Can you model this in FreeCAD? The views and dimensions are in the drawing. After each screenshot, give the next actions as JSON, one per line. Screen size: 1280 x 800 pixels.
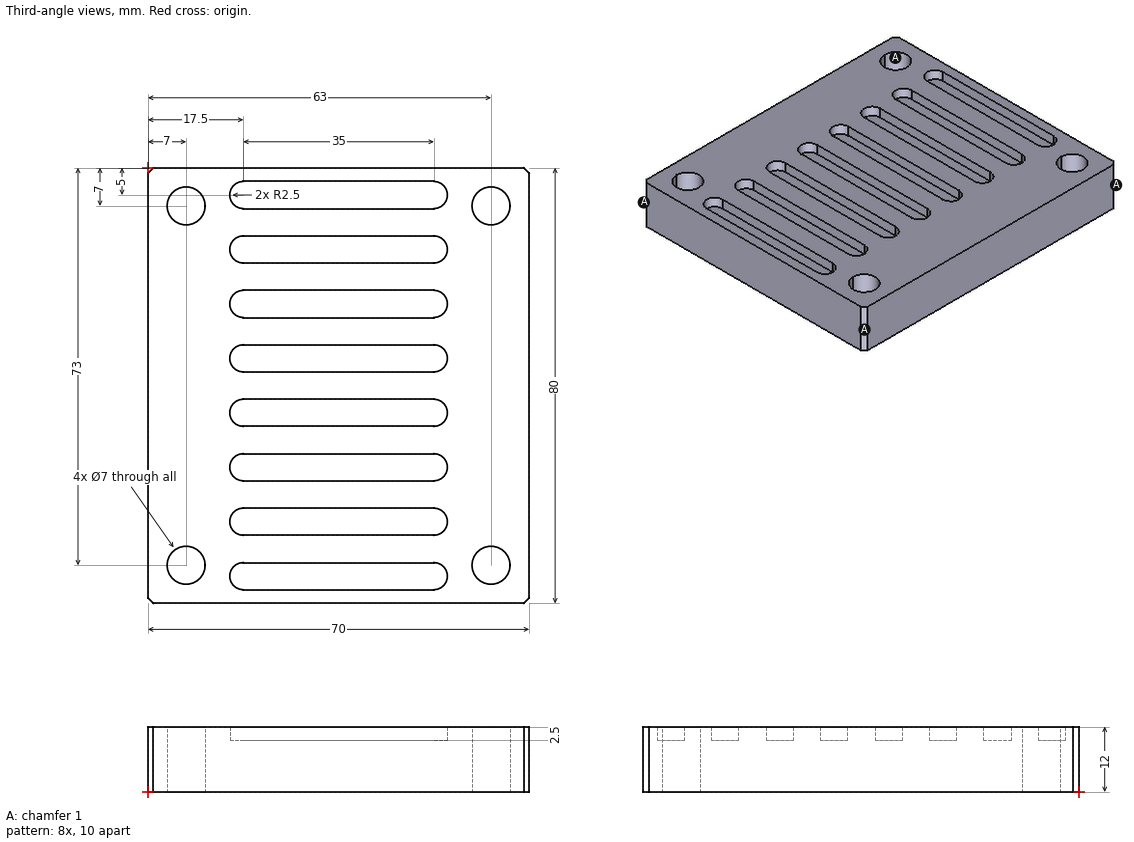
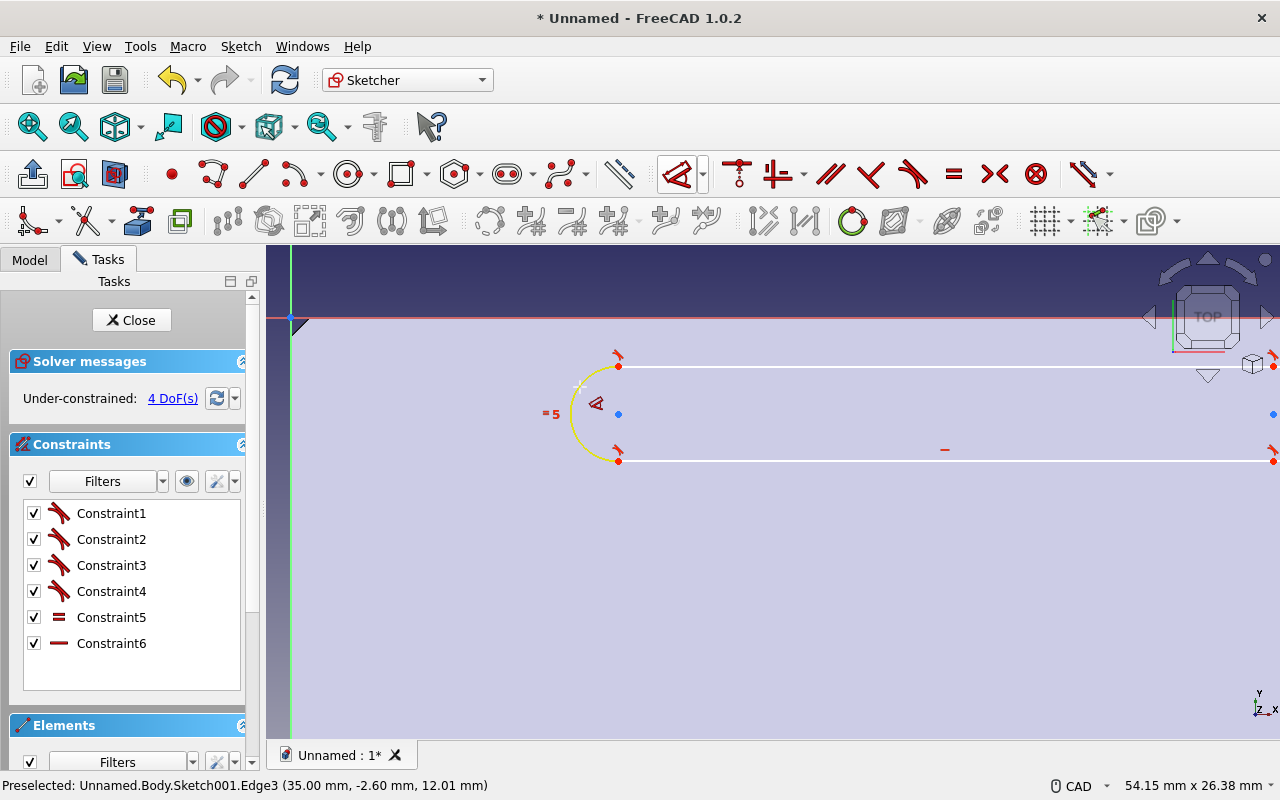
{"action": "left_click", "coordinate": [580, 386]}
{"action": "left_click", "coordinate": [554, 367]}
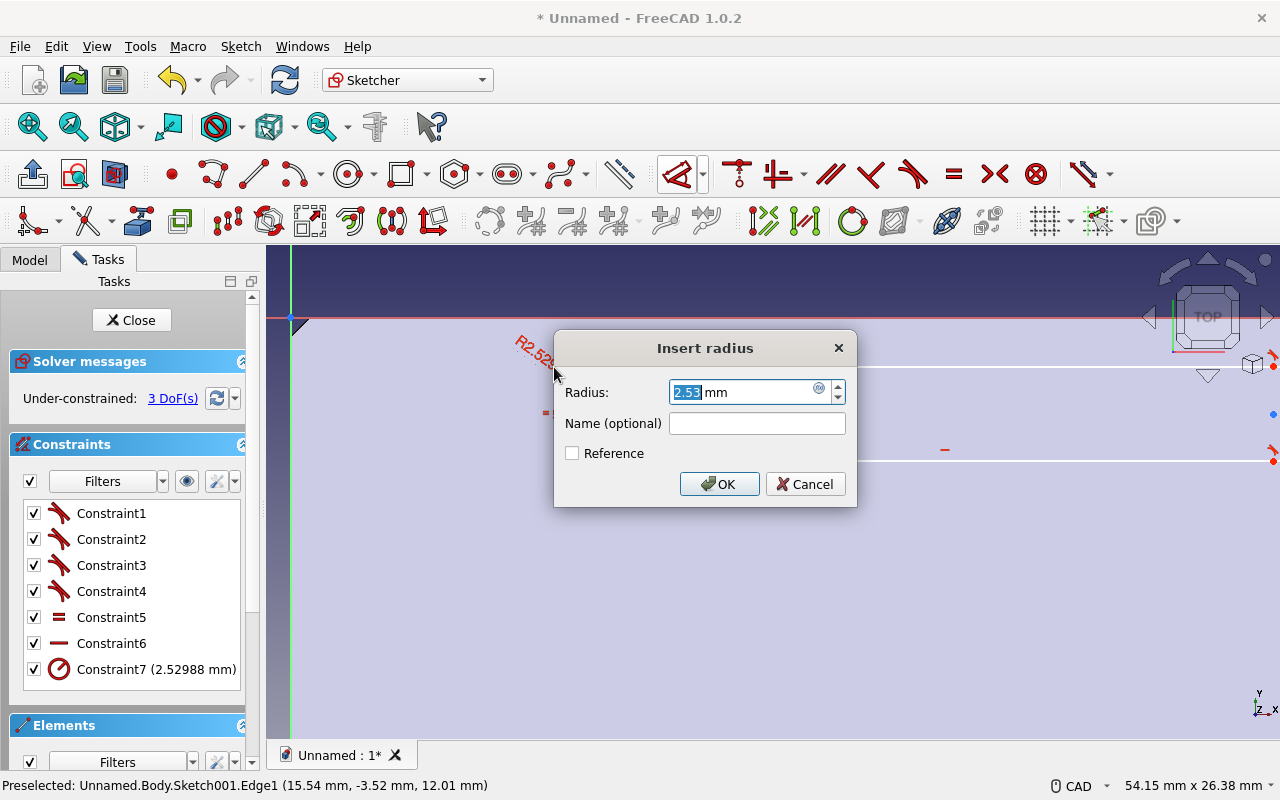
{"action": "type", "text": "2.5"}
{"action": "key", "text": "Return"}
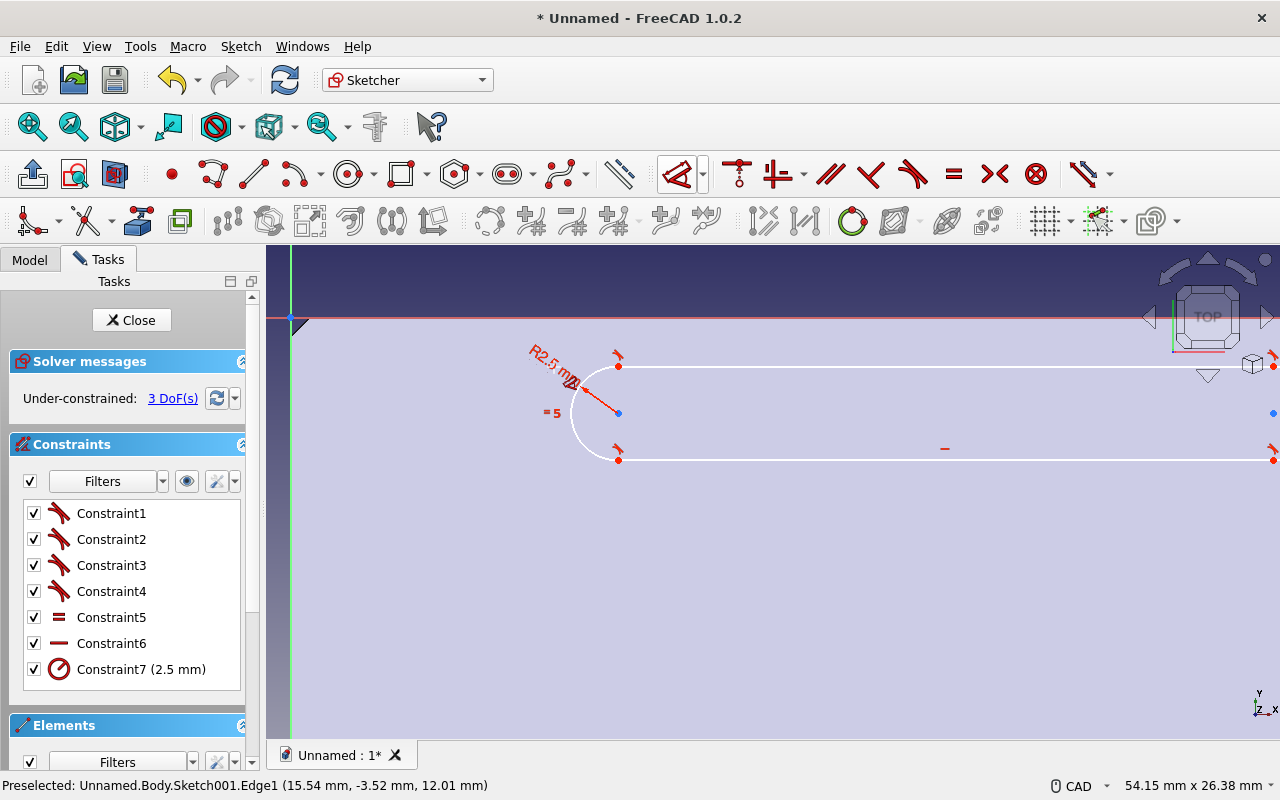
{"action": "left_click", "coordinate": [815, 367]}
{"action": "left_click", "coordinate": [867, 333]}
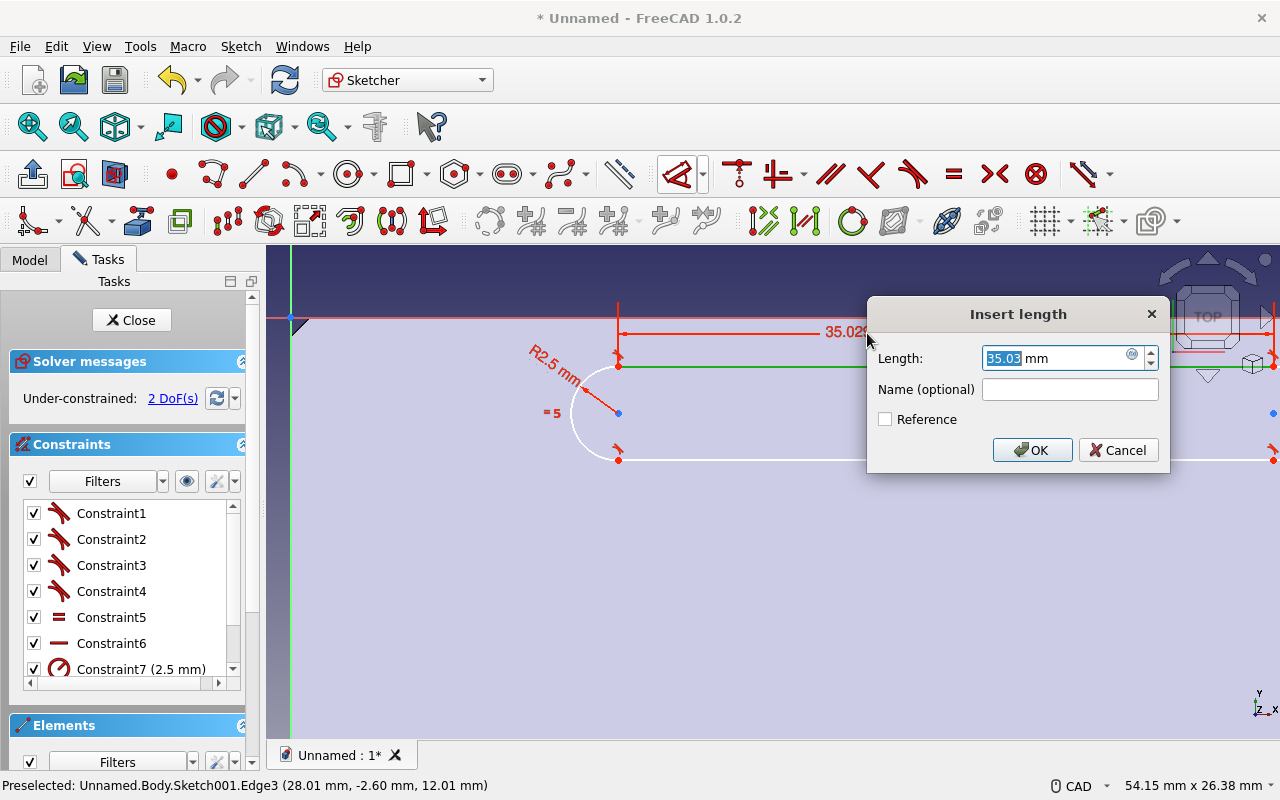
{"action": "type", "text": "35"}
{"action": "key", "text": "Return"}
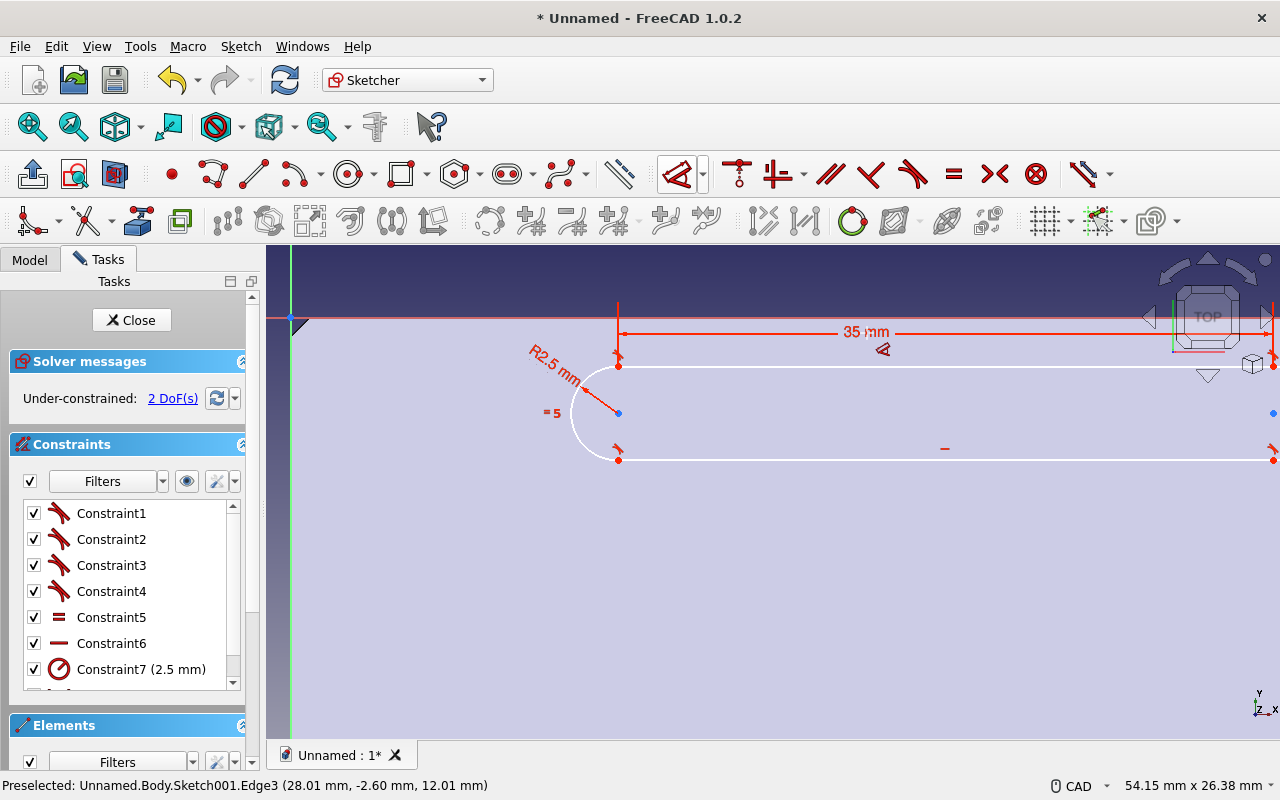
{"action": "left_click", "coordinate": [618, 414]}
{"action": "left_click", "coordinate": [652, 344]}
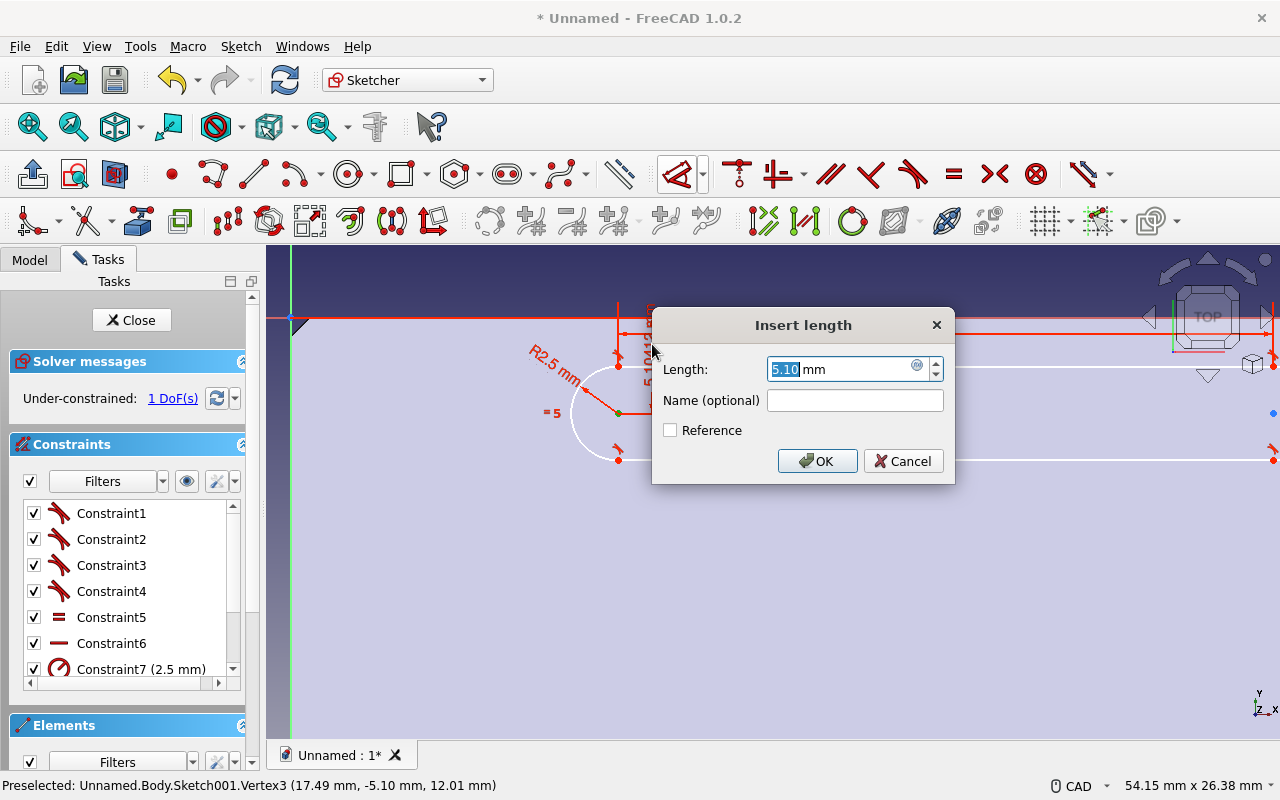
{"action": "type", "text": "5"}
{"action": "key", "text": "Return"}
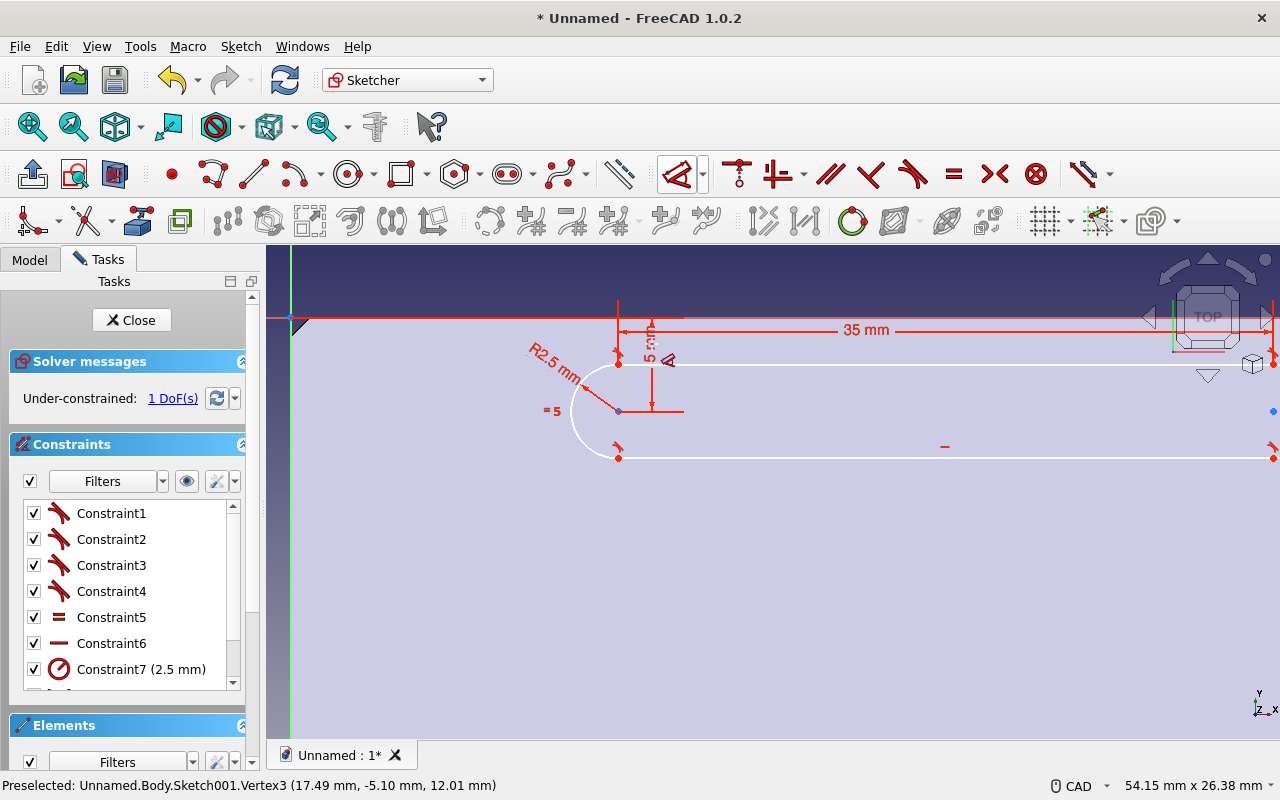
{"action": "left_click", "coordinate": [618, 365]}
{"action": "left_click", "coordinate": [456, 284]}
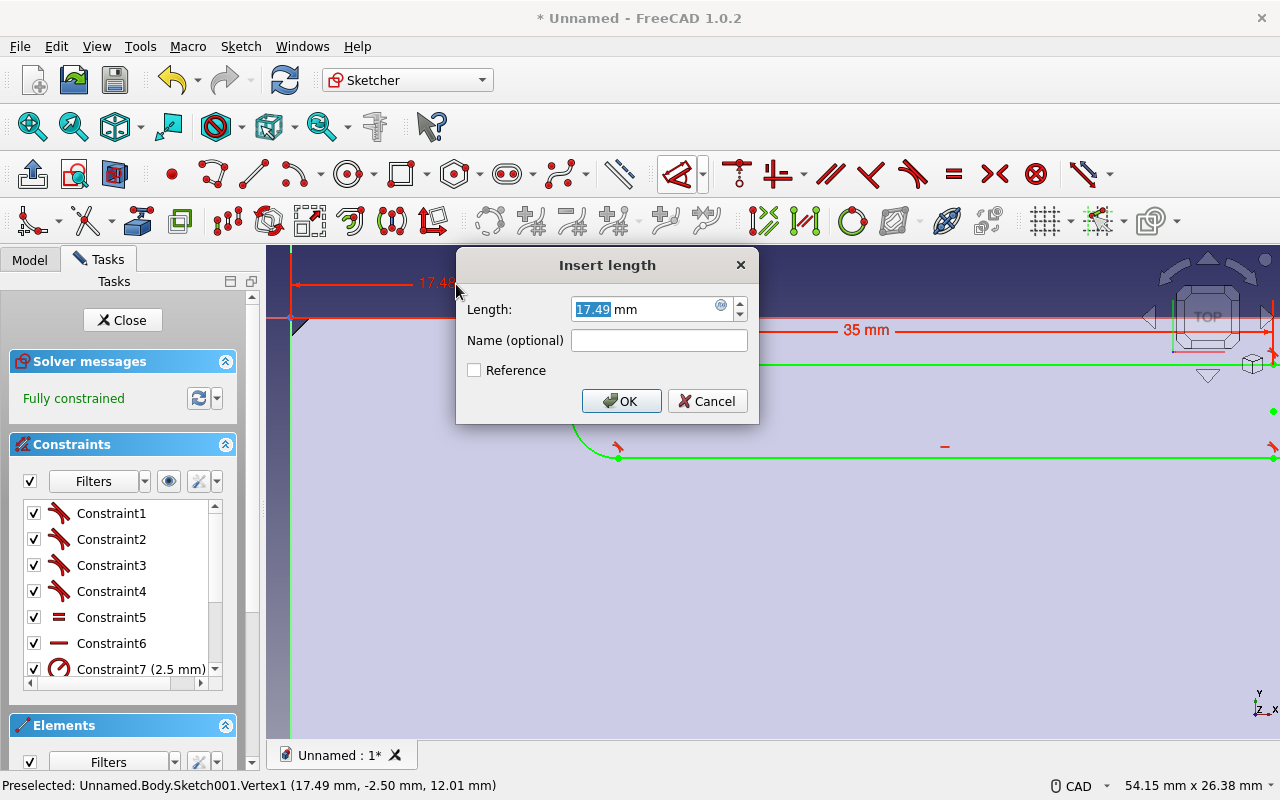
{"action": "type", "text": "17.5"}
{"action": "key", "text": "Return"}
{"action": "key", "text": "Escape"}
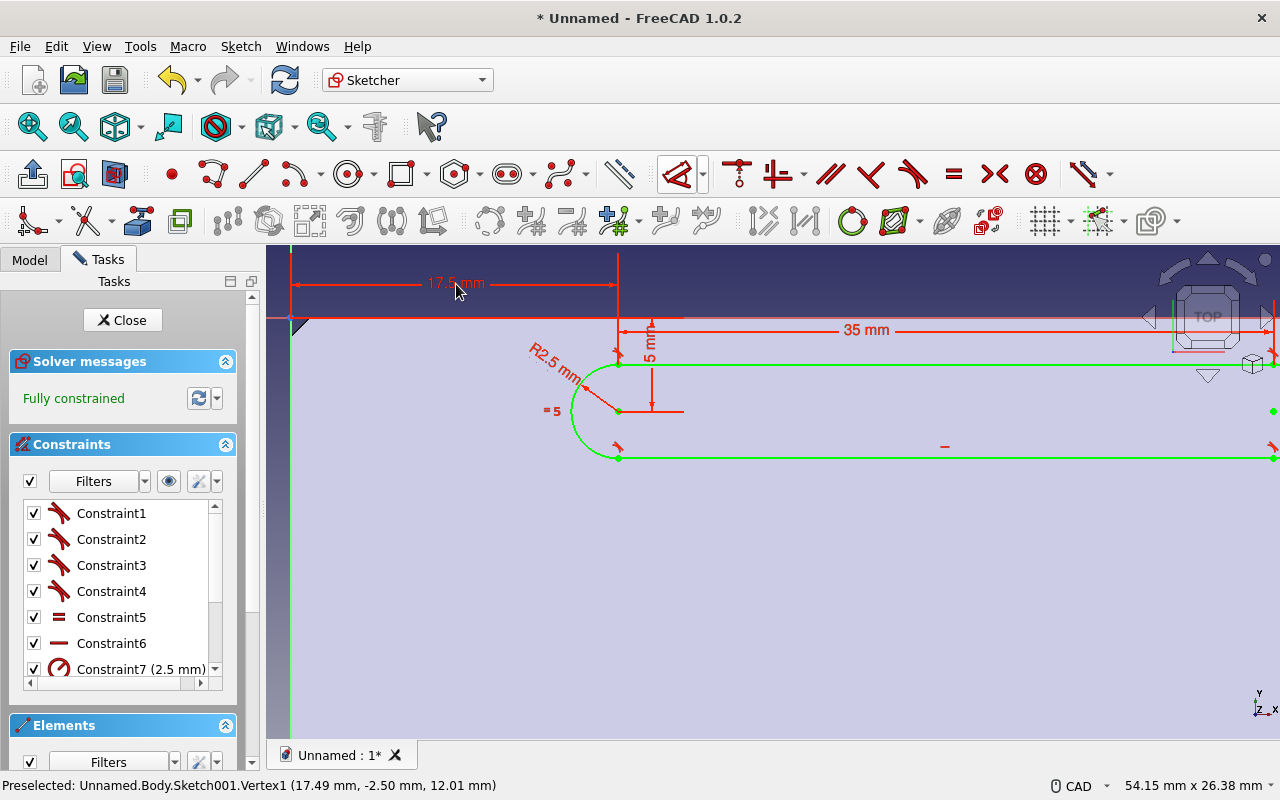
{"action": "left_click", "coordinate": [123, 320]}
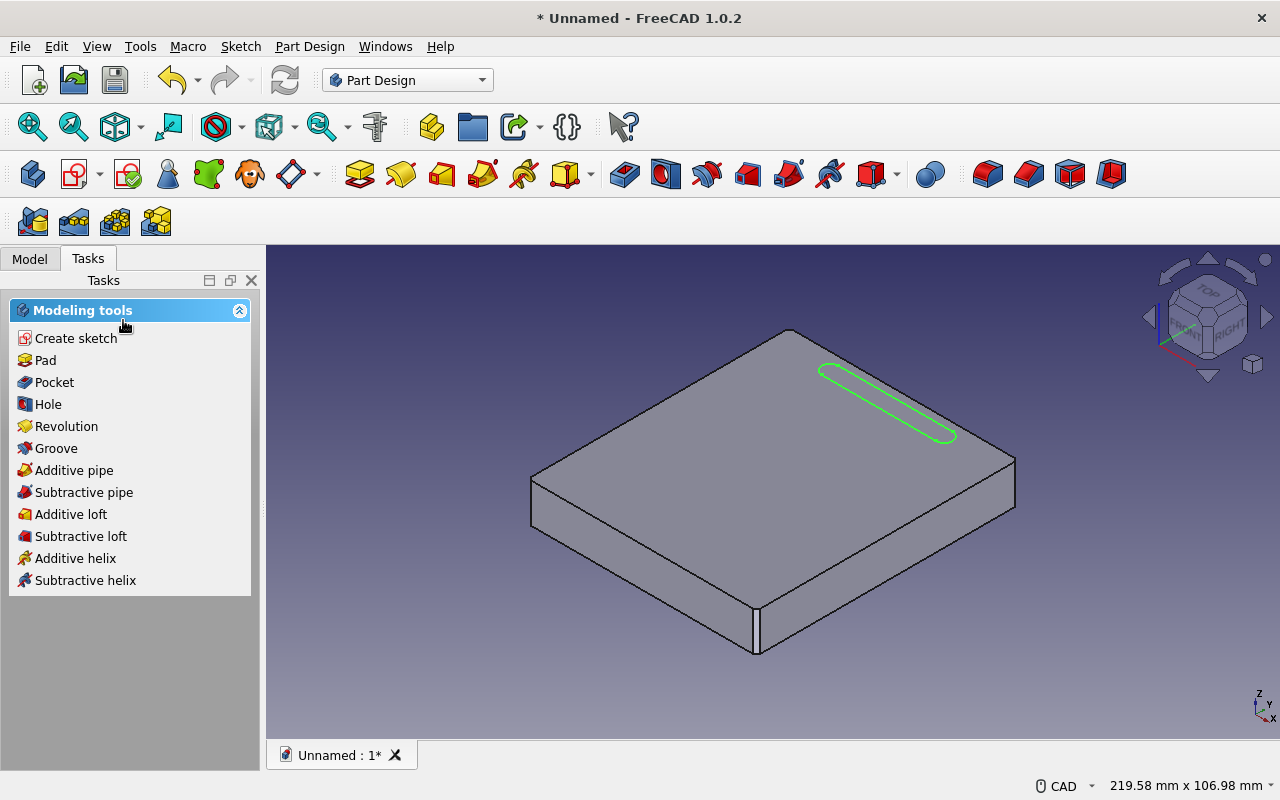
{"action": "left_click", "coordinate": [625, 174]}